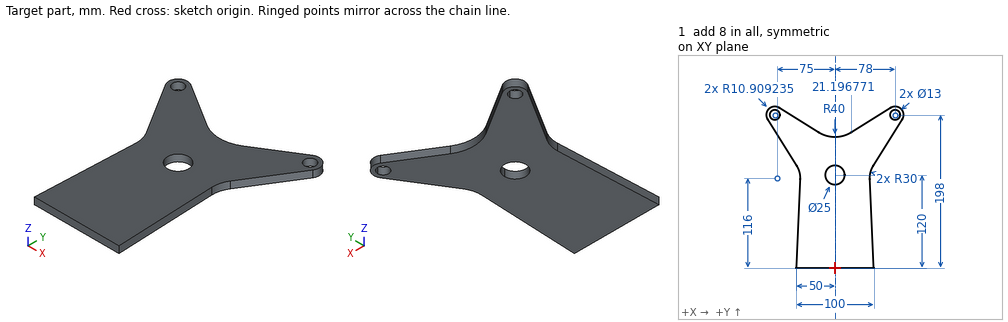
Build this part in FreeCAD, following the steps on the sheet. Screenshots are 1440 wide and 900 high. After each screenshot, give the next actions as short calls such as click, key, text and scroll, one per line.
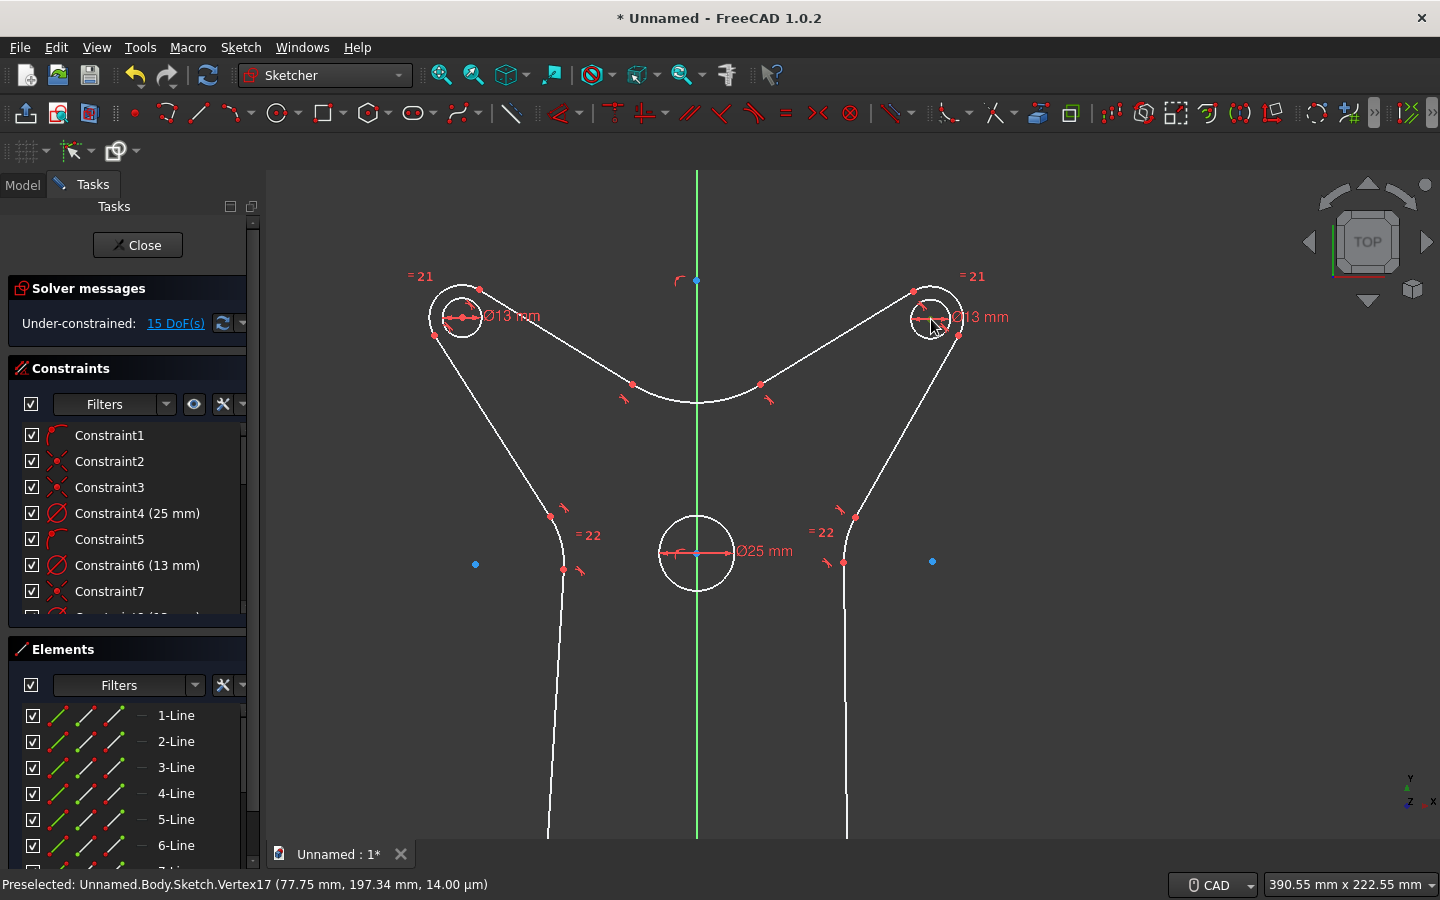
click(462, 318)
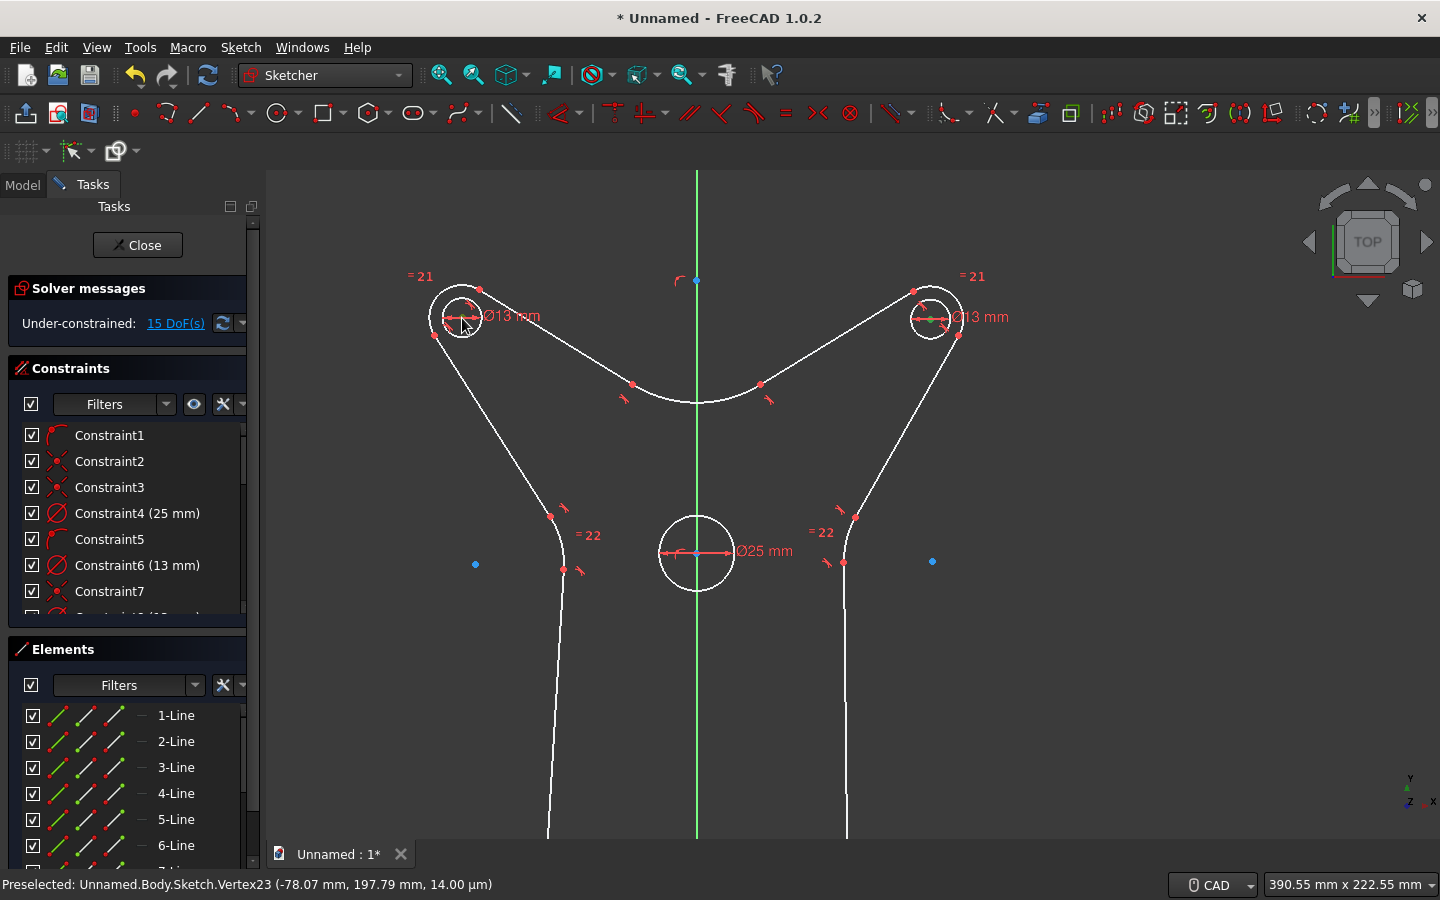
click(697, 767)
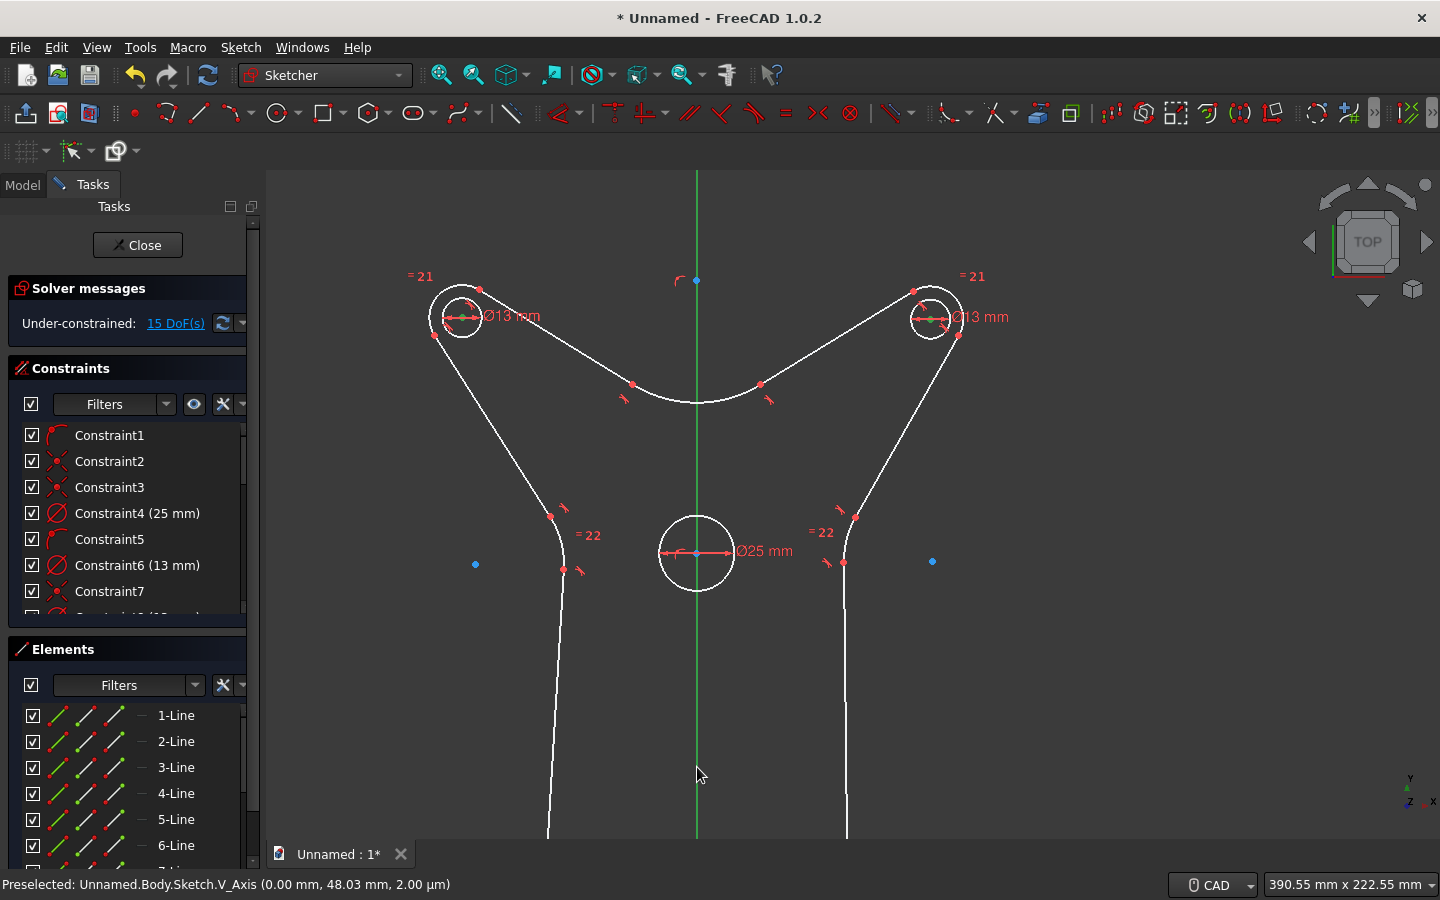
click(818, 114)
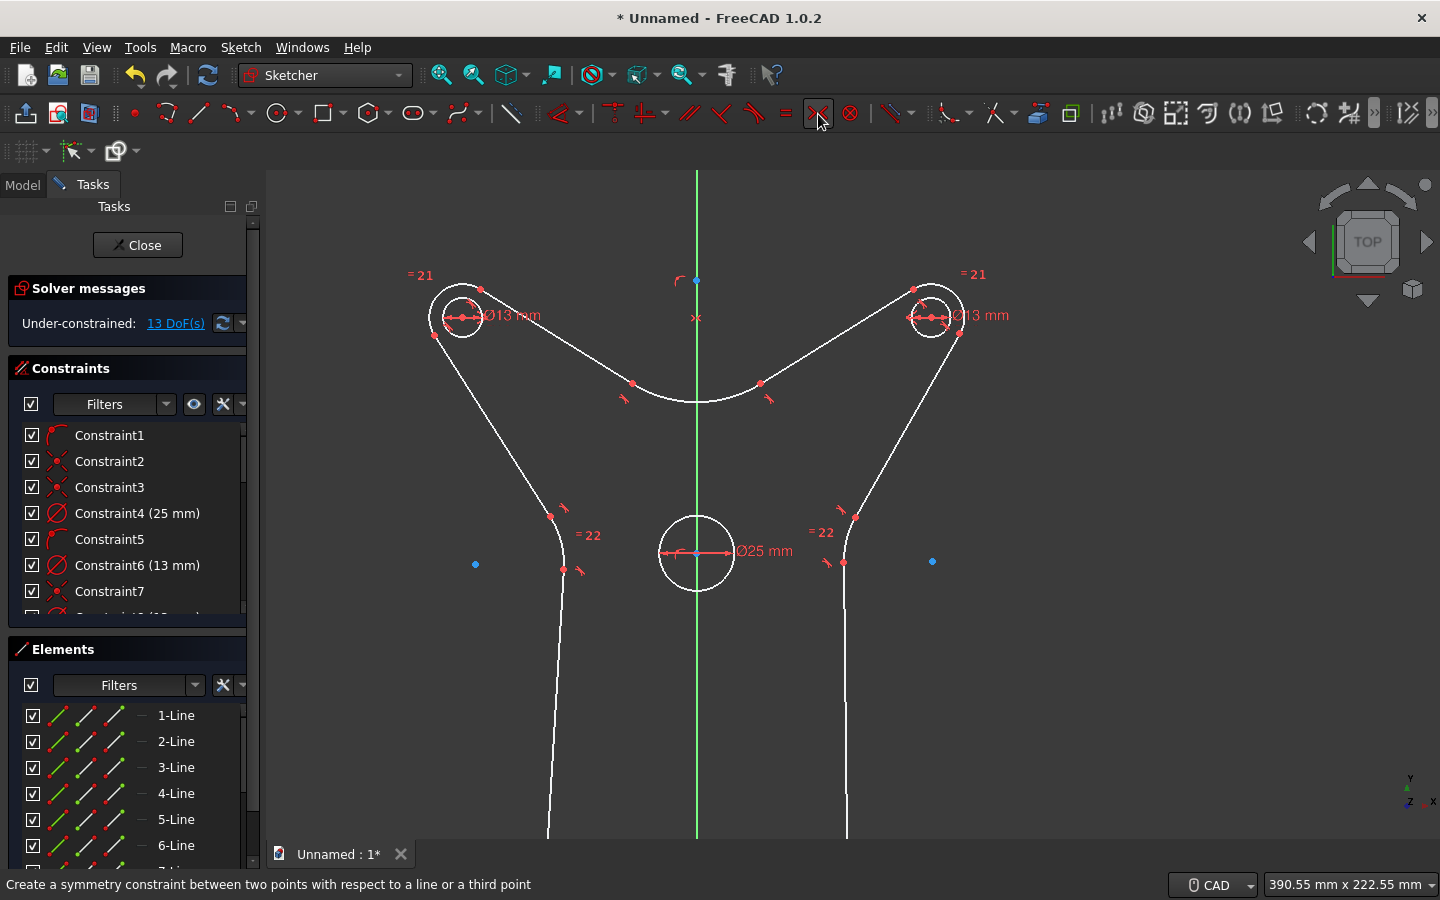
click(476, 564)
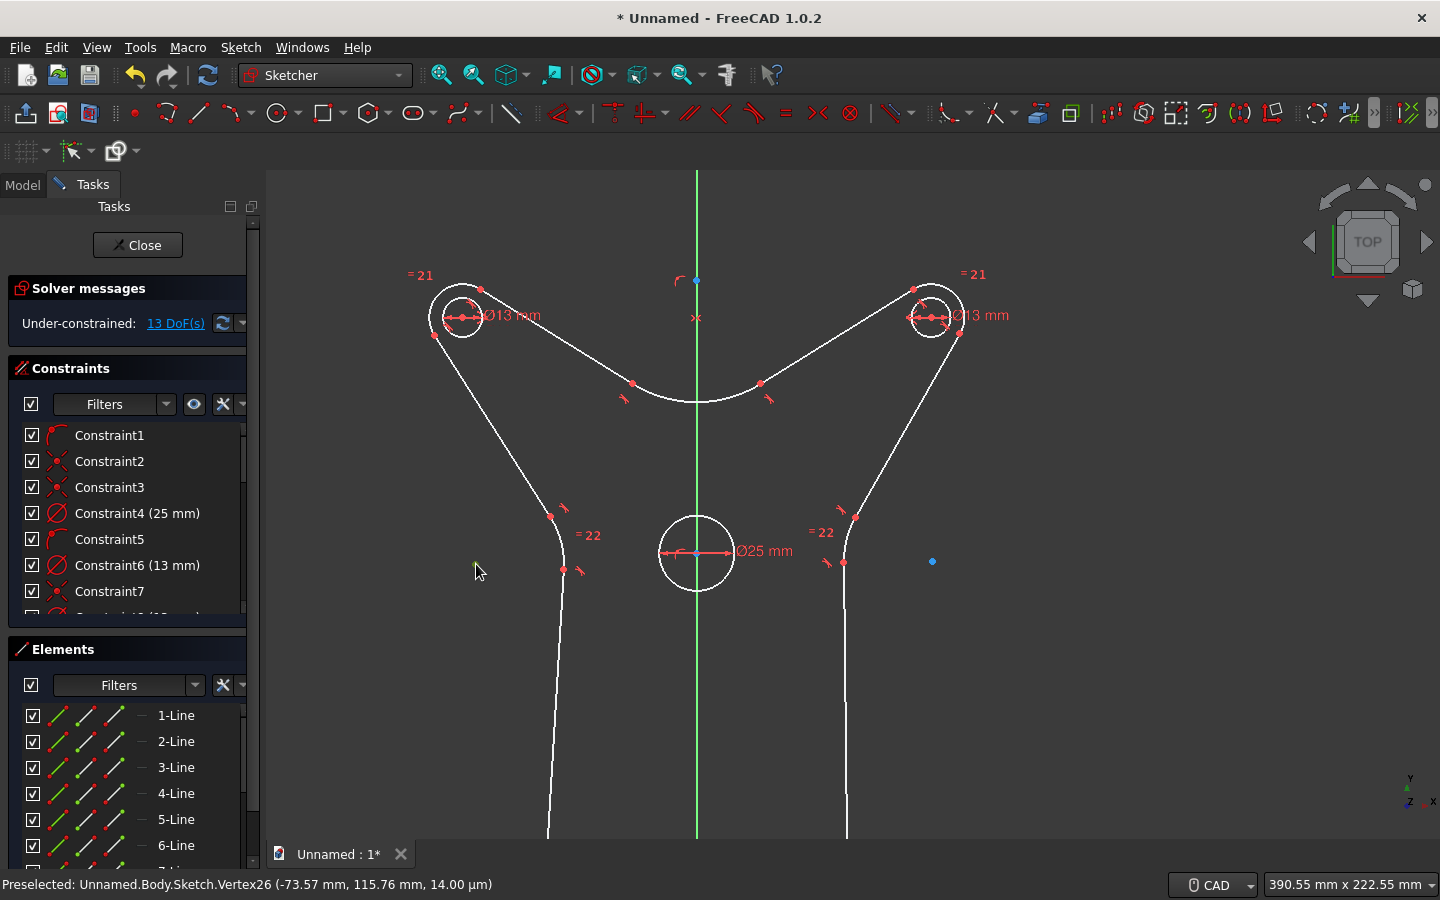
click(932, 561)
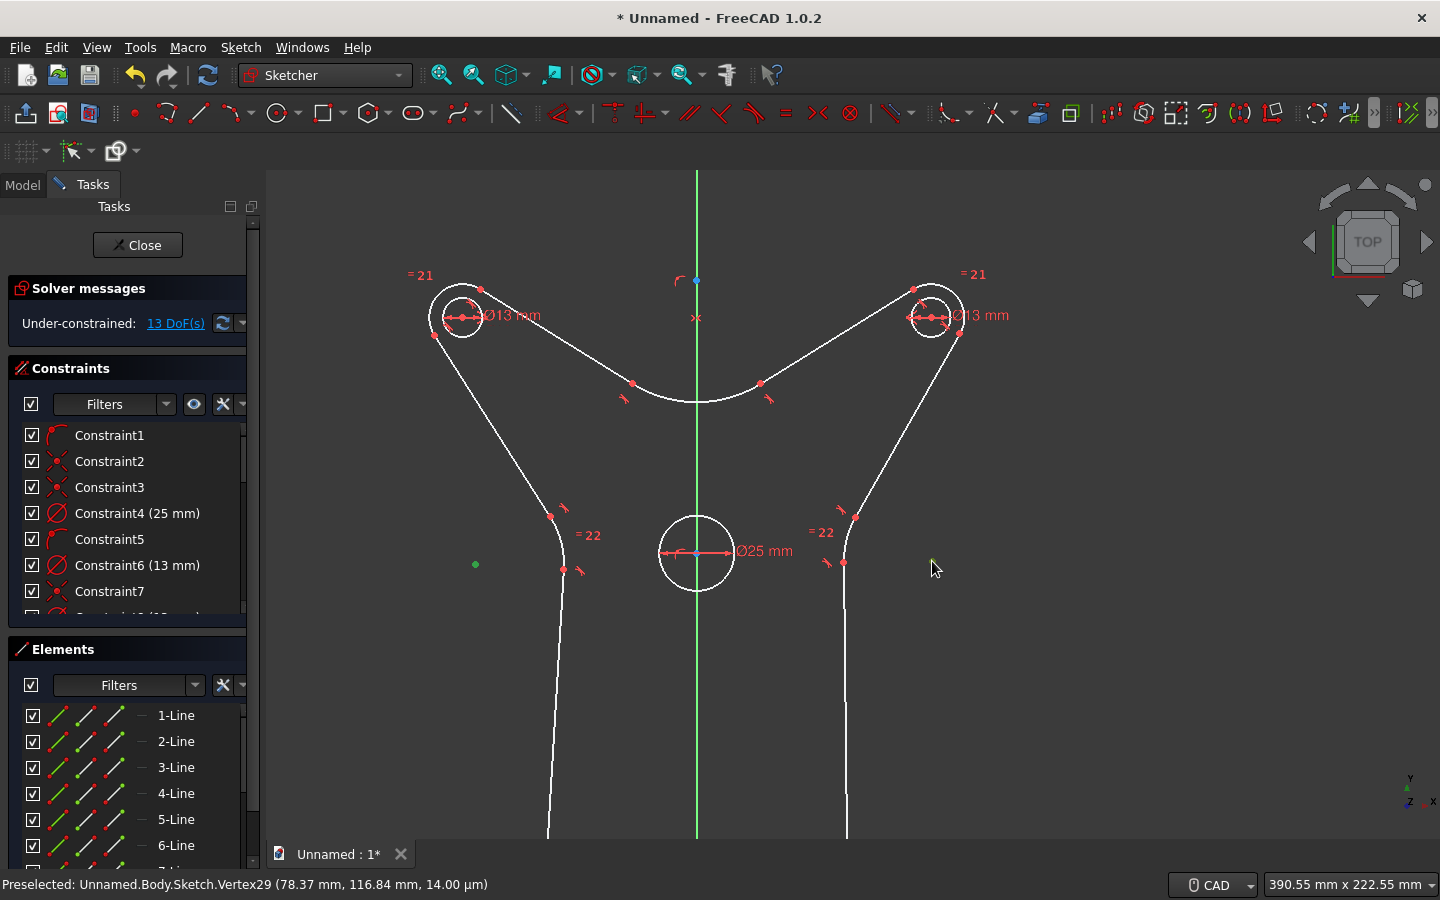
click(697, 767)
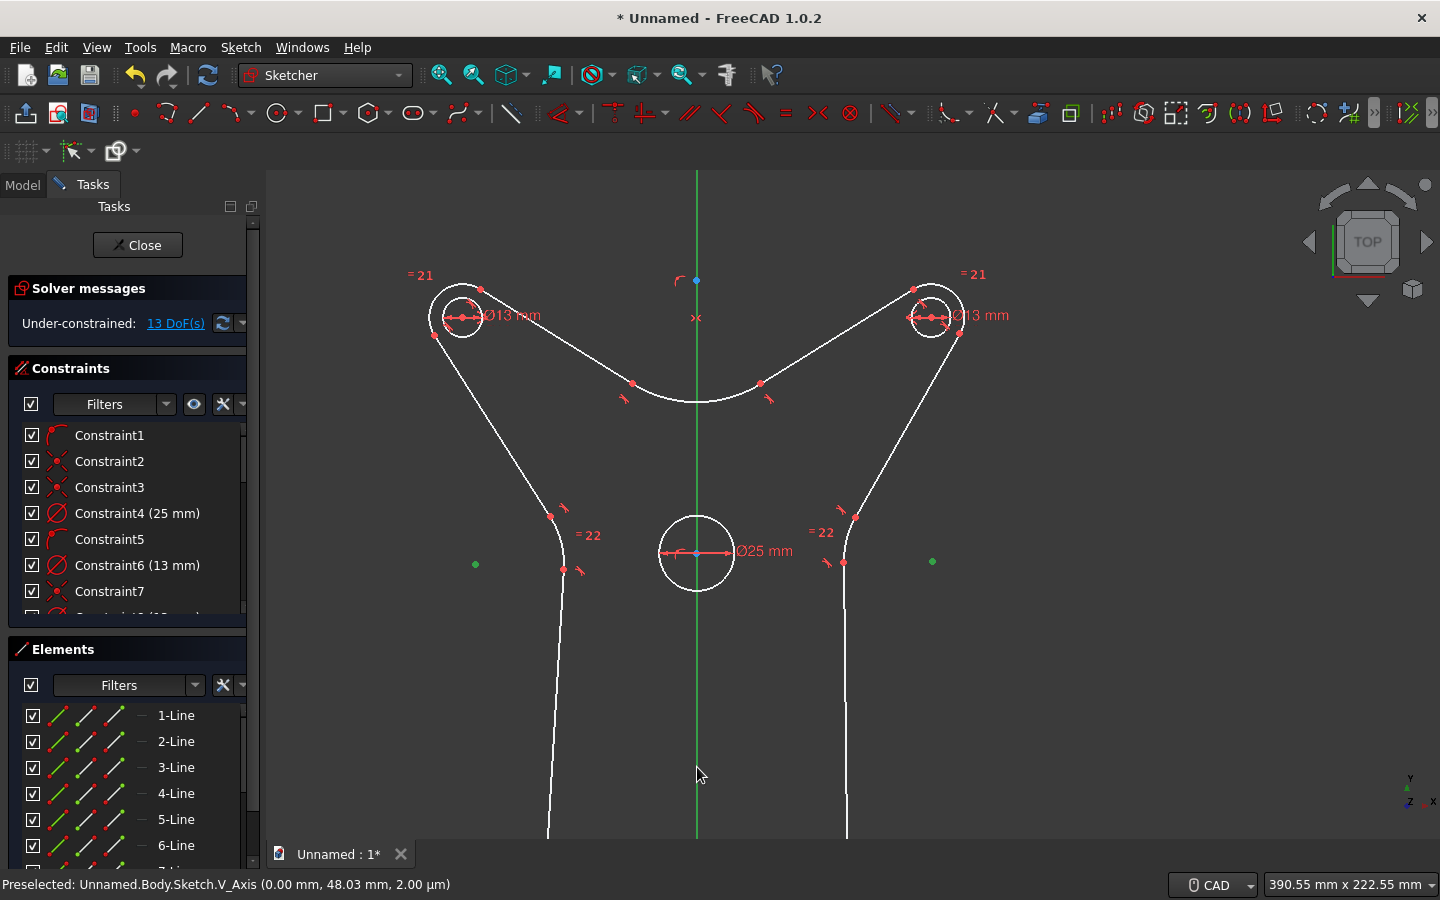
click(818, 114)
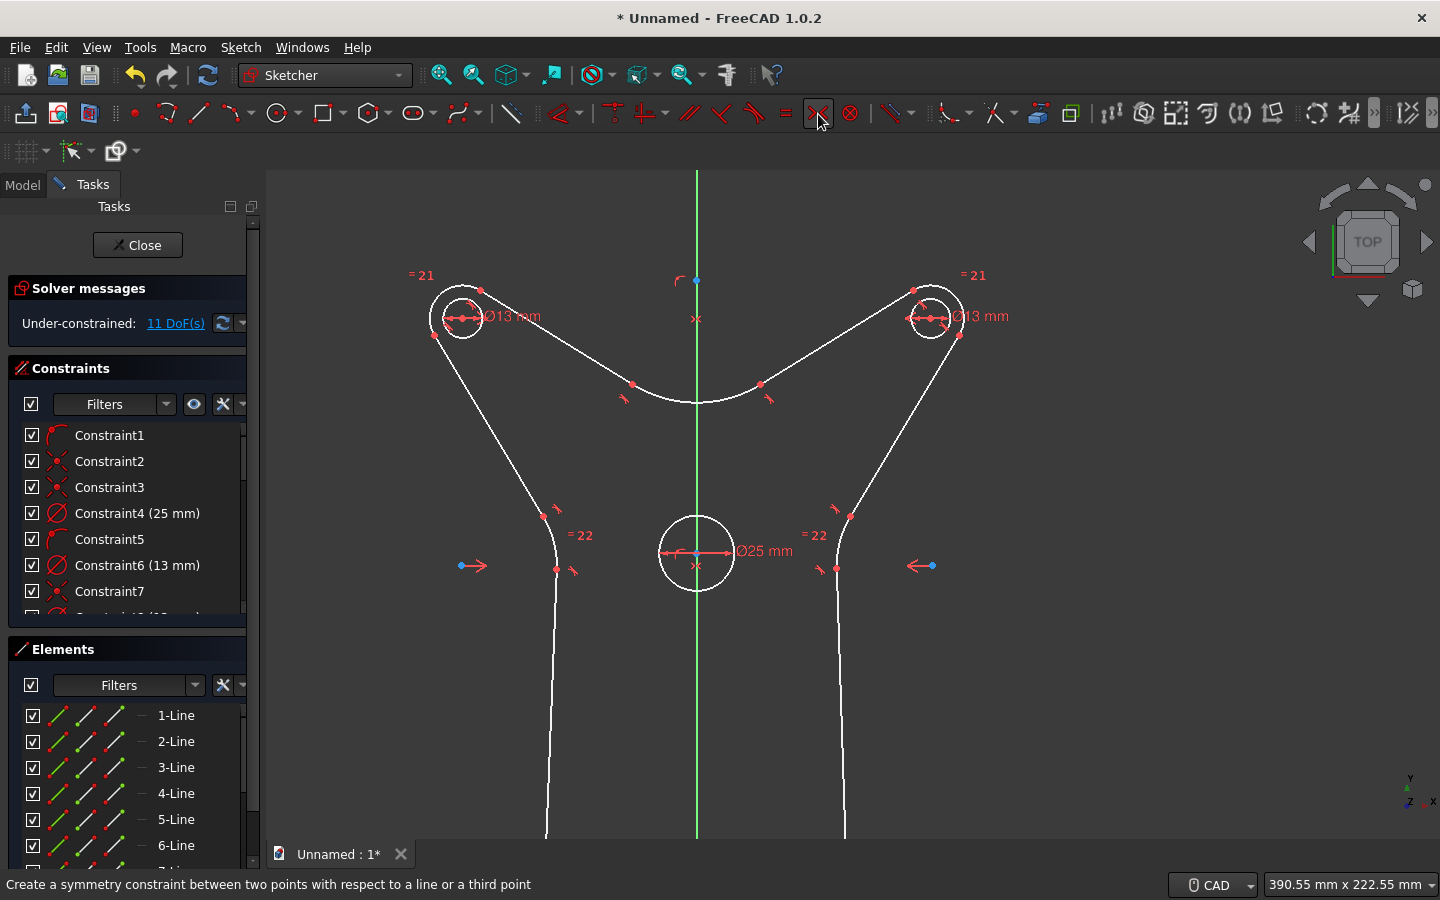
click(558, 114)